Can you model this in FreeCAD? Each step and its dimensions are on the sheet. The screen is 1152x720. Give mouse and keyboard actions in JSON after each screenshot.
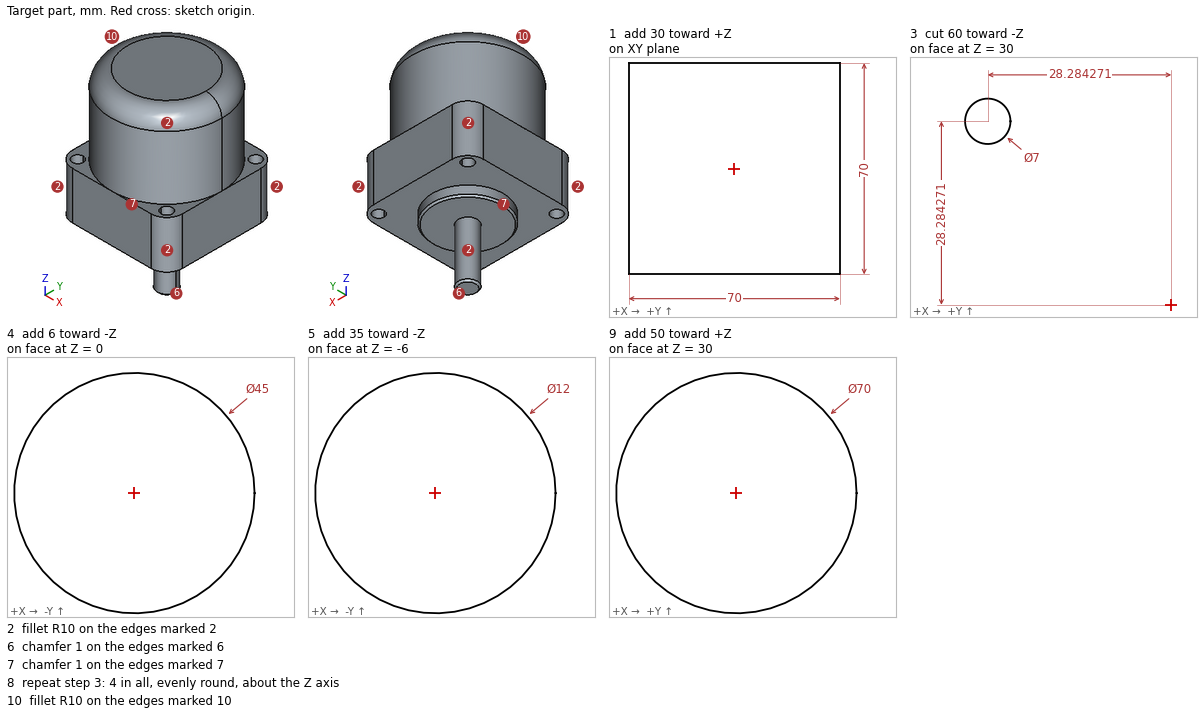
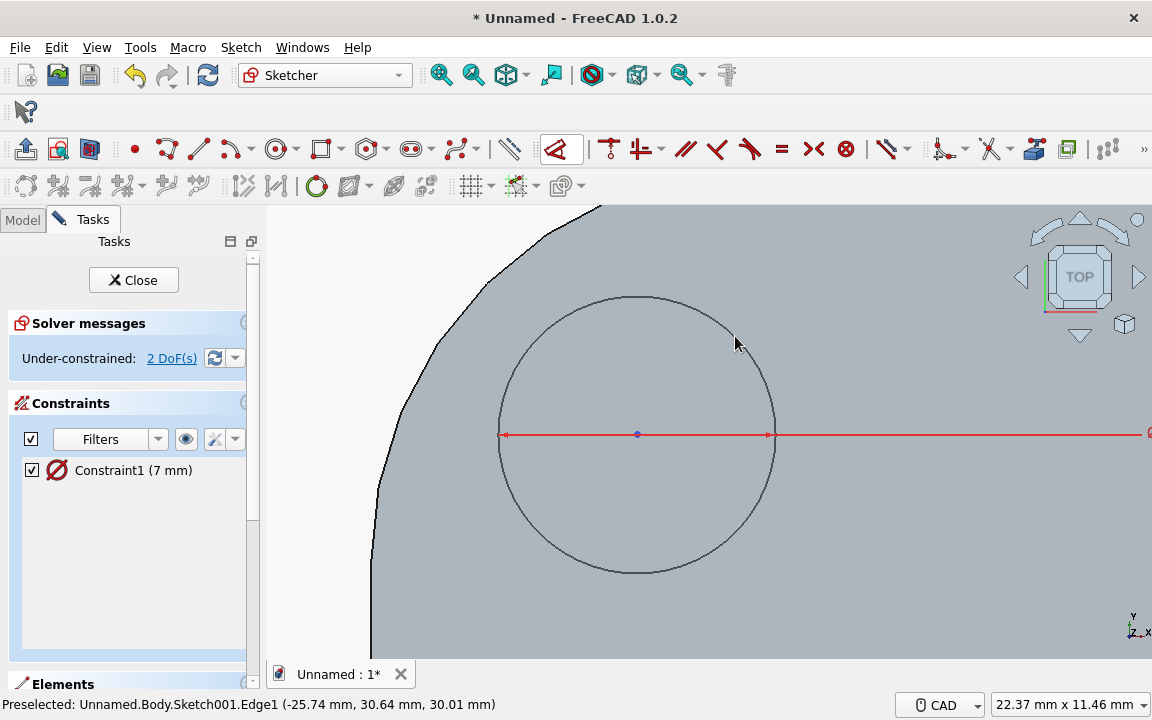
{"action": "key", "text": "d"}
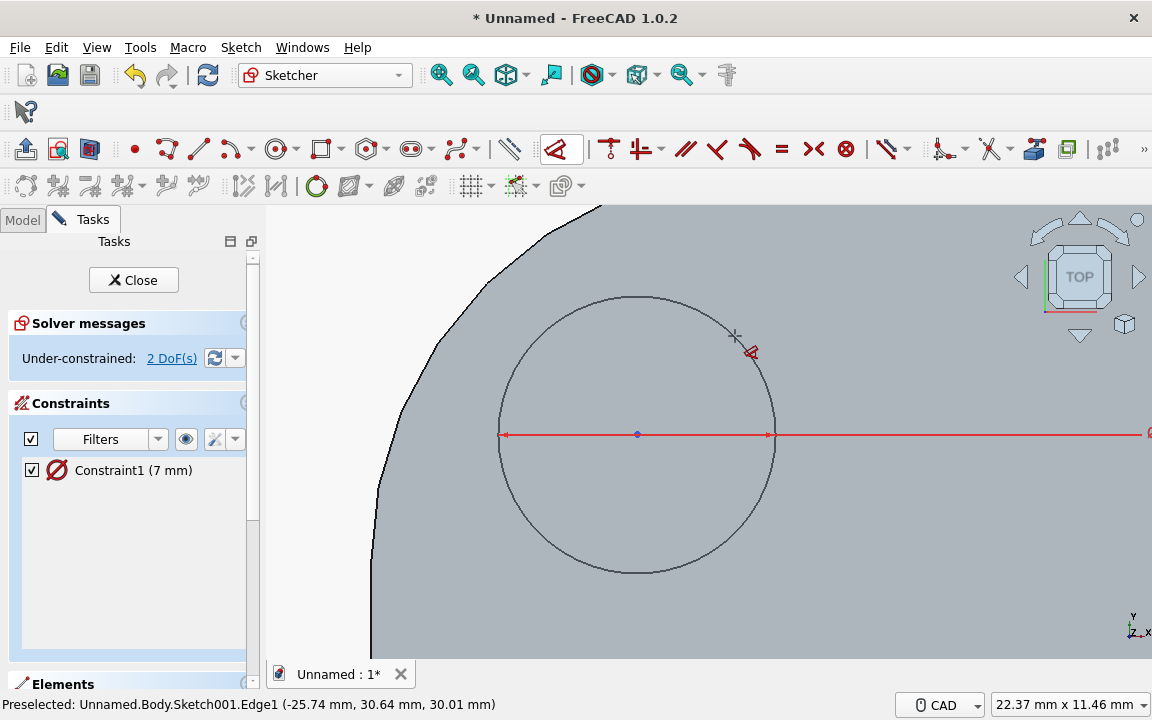
{"action": "left_click", "coordinate": [637, 435]}
{"action": "left_click", "coordinate": [812, 401]}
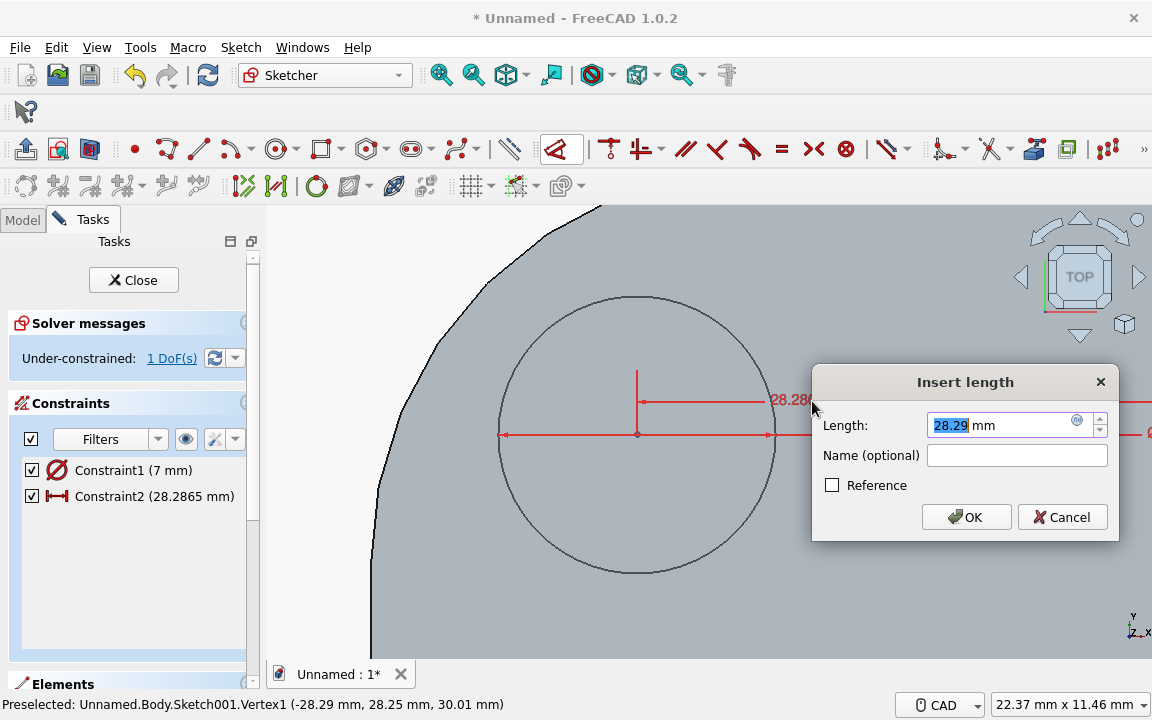
{"action": "type", "text": "28.284271"}
{"action": "key", "text": "Return"}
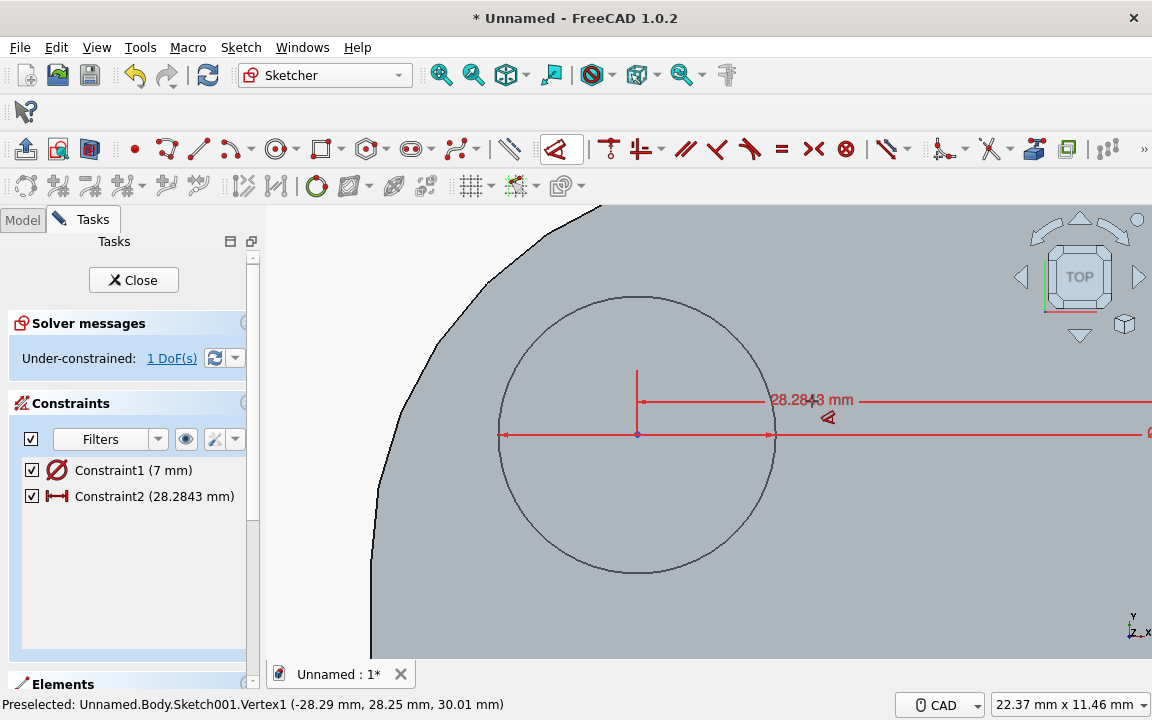
{"action": "left_click", "coordinate": [637, 435]}
{"action": "left_click", "coordinate": [603, 533]}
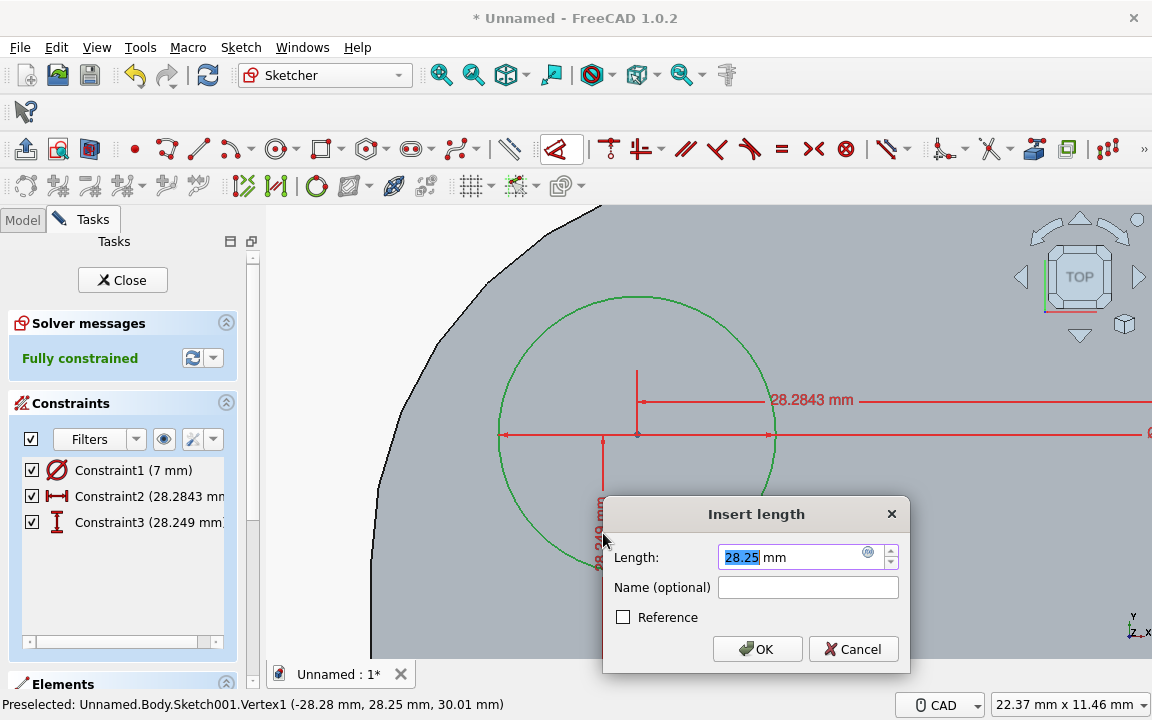
{"action": "type", "text": "28.284271"}
{"action": "key", "text": "Return"}
{"action": "key", "text": "Escape"}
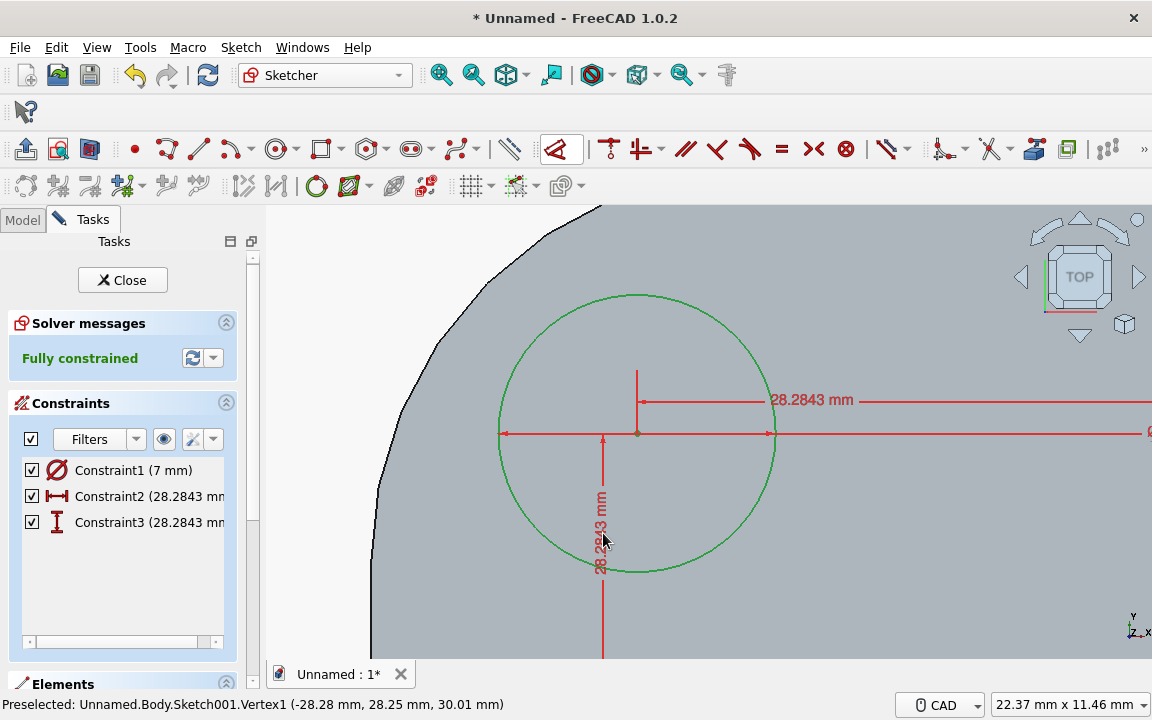
{"action": "left_click", "coordinate": [123, 280]}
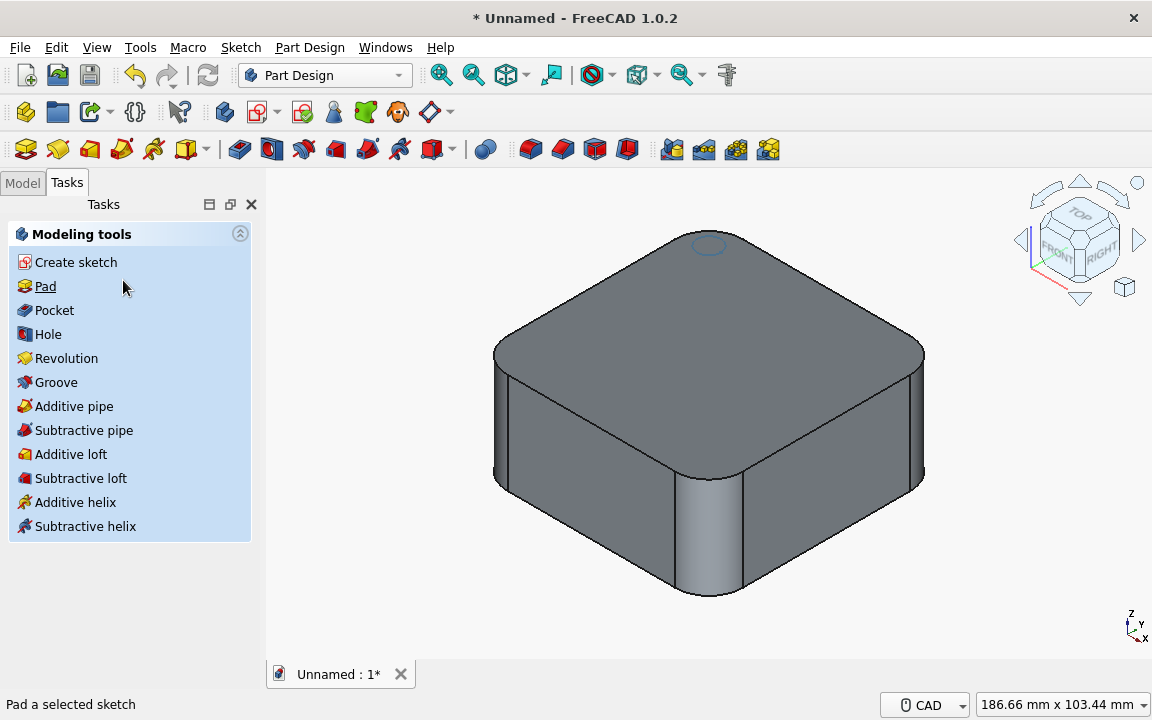
{"action": "left_click", "coordinate": [240, 150]}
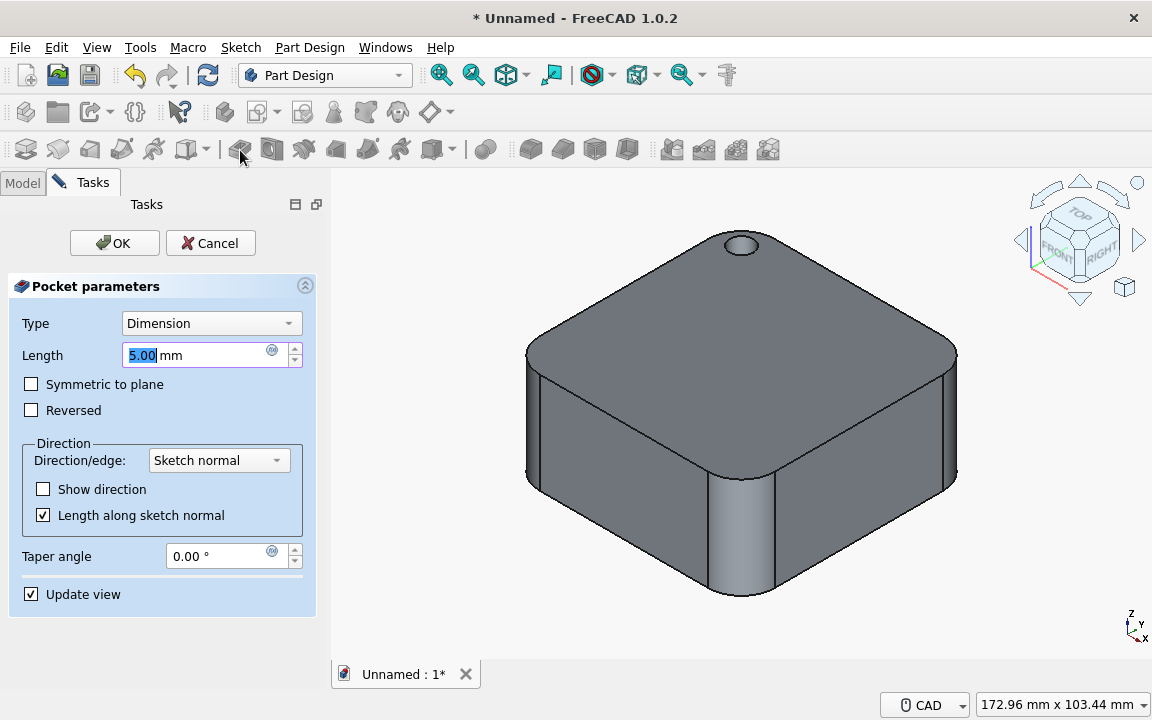
{"action": "type", "text": "60"}
{"action": "key", "text": "Tab"}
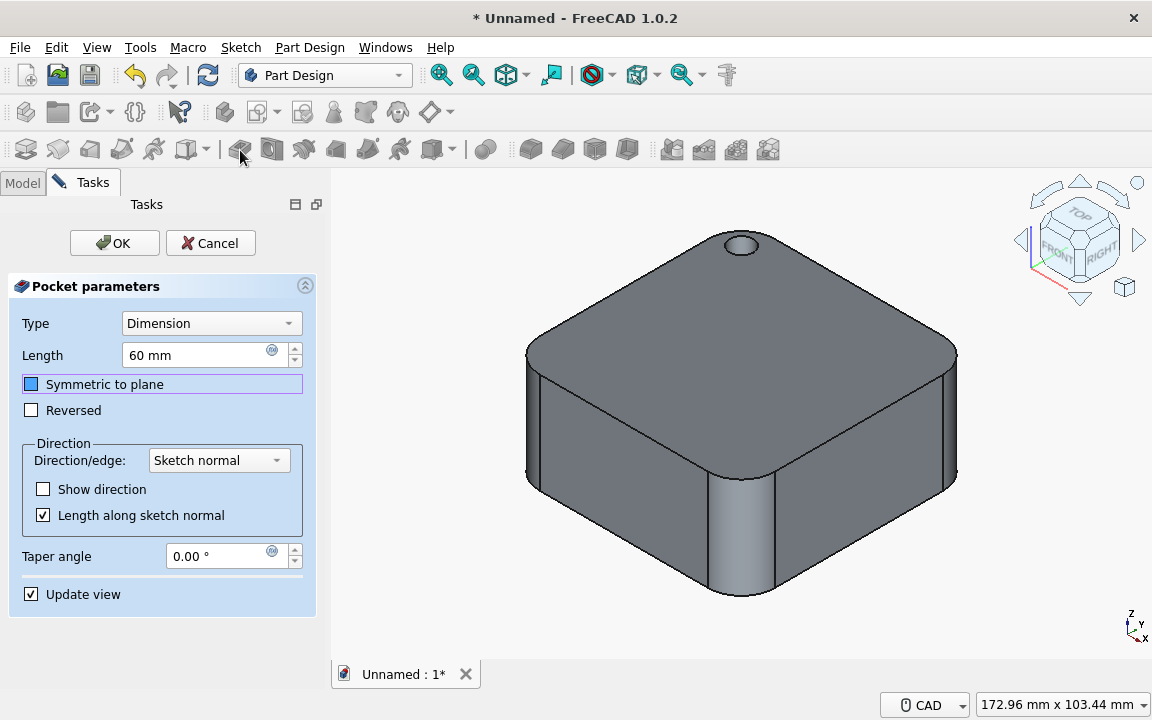
{"action": "left_click", "coordinate": [115, 243]}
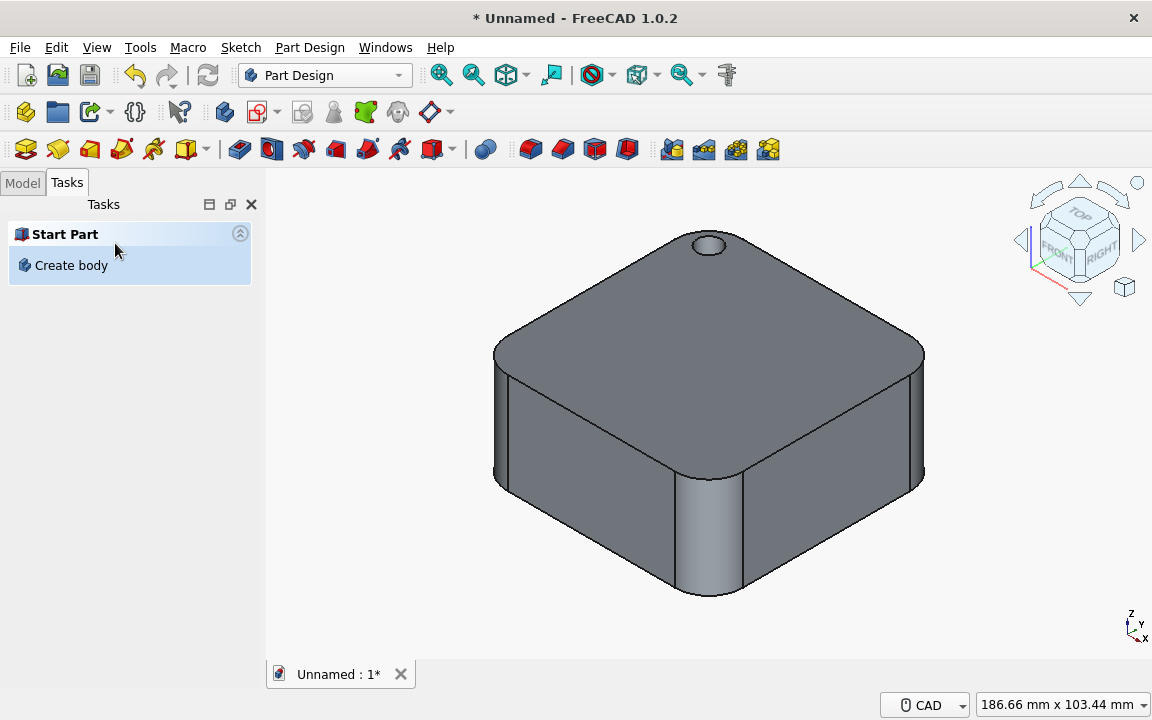
{"action": "key", "text": "5"}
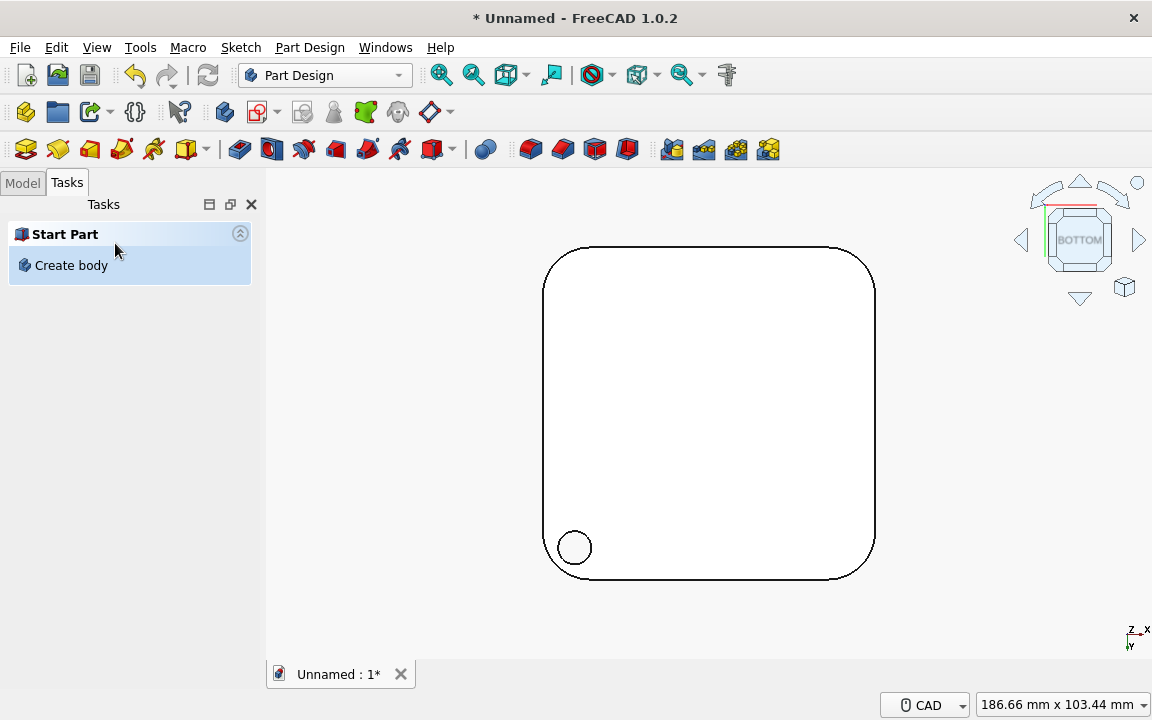
{"action": "left_click", "coordinate": [709, 413]}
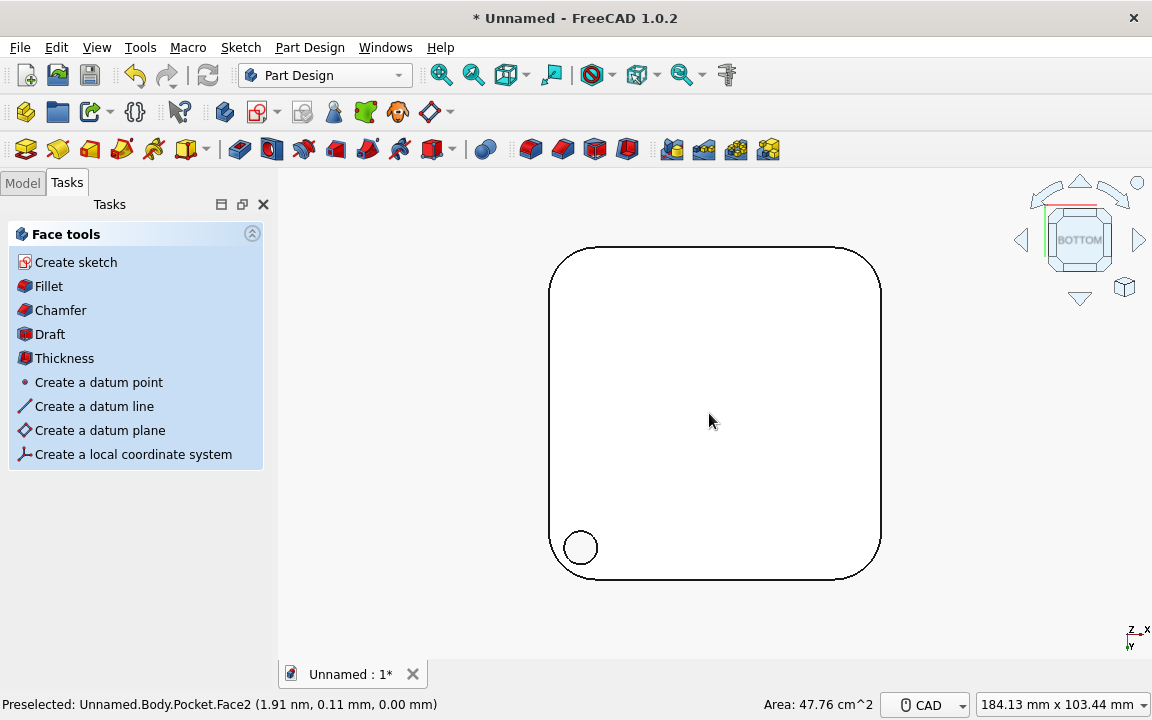
{"action": "left_click", "coordinate": [258, 112]}